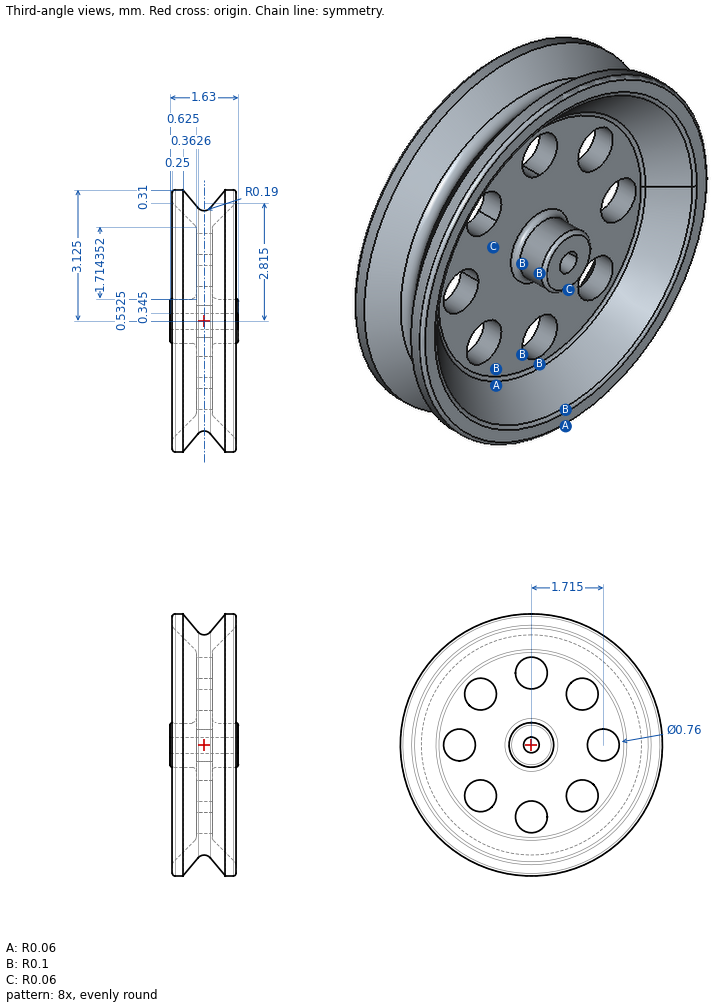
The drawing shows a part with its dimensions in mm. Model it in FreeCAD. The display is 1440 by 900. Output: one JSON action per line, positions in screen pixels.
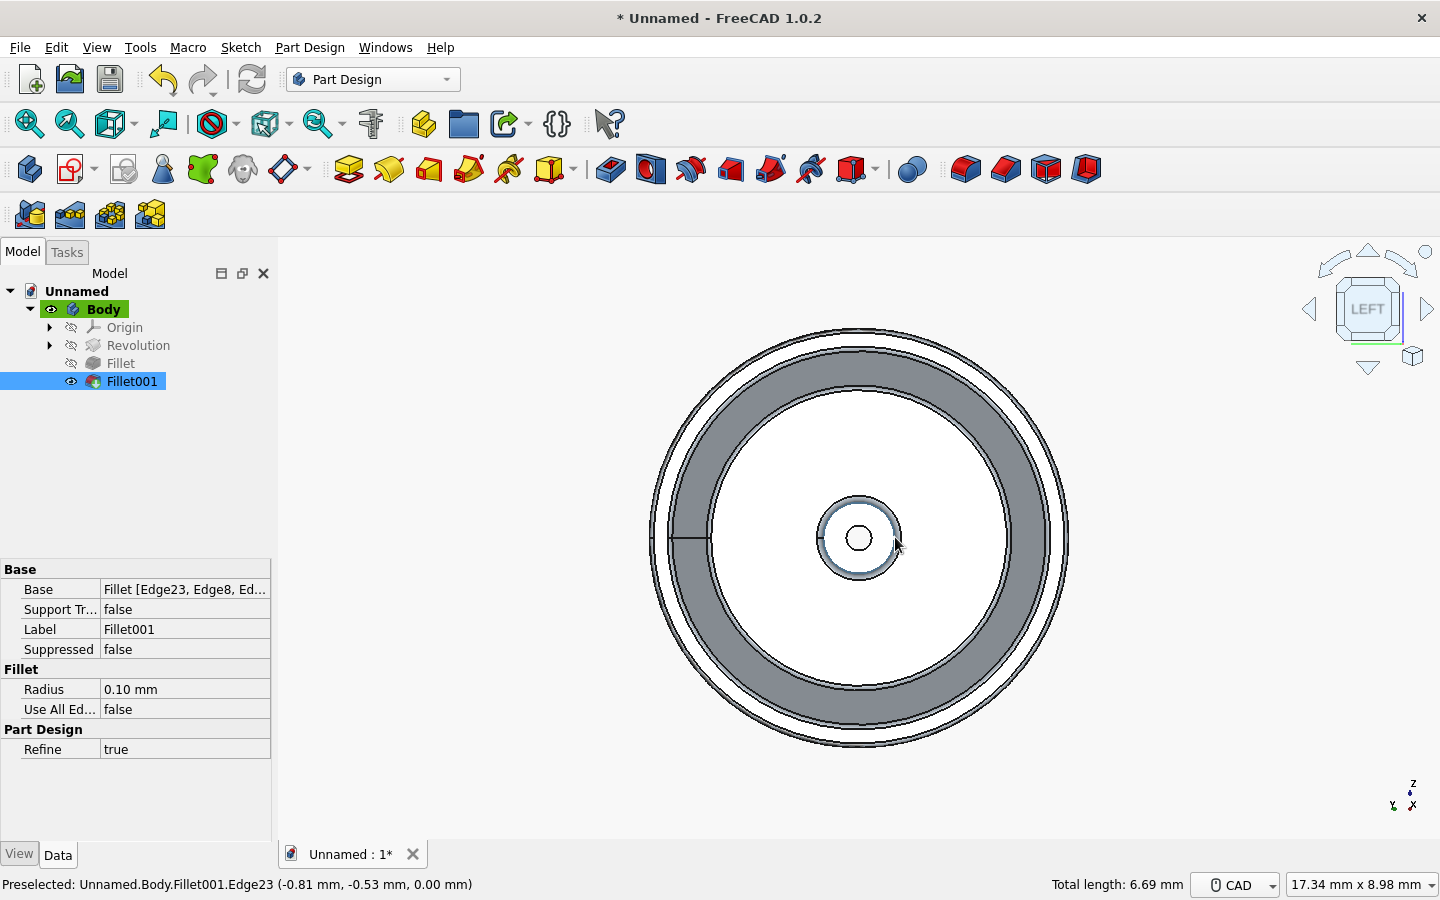
{"action": "left_click", "coordinate": [966, 170]}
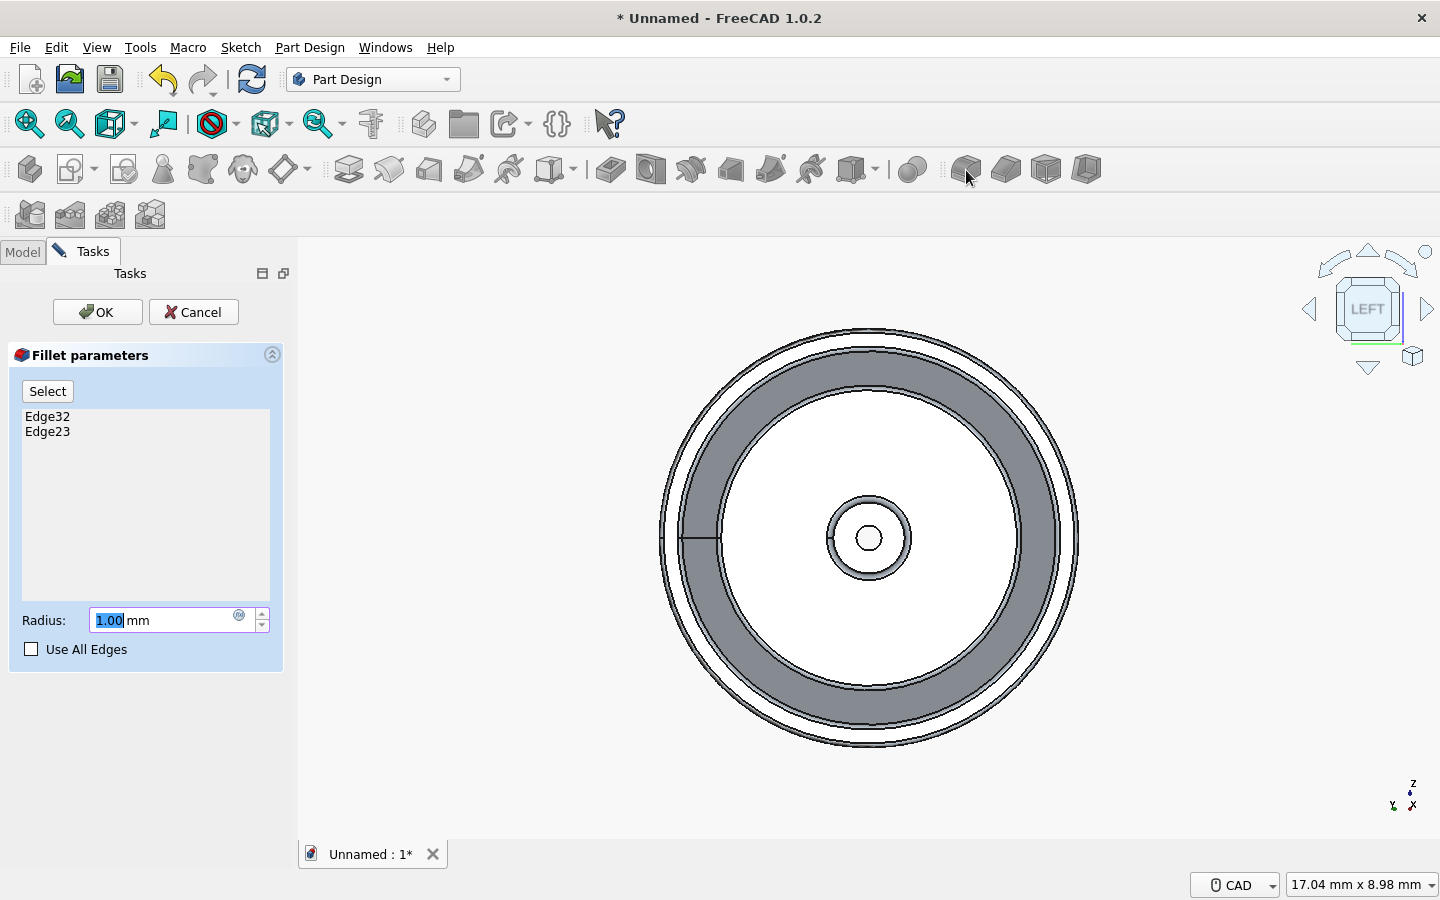
{"action": "type", "text": "0.06"}
{"action": "key", "text": "Tab"}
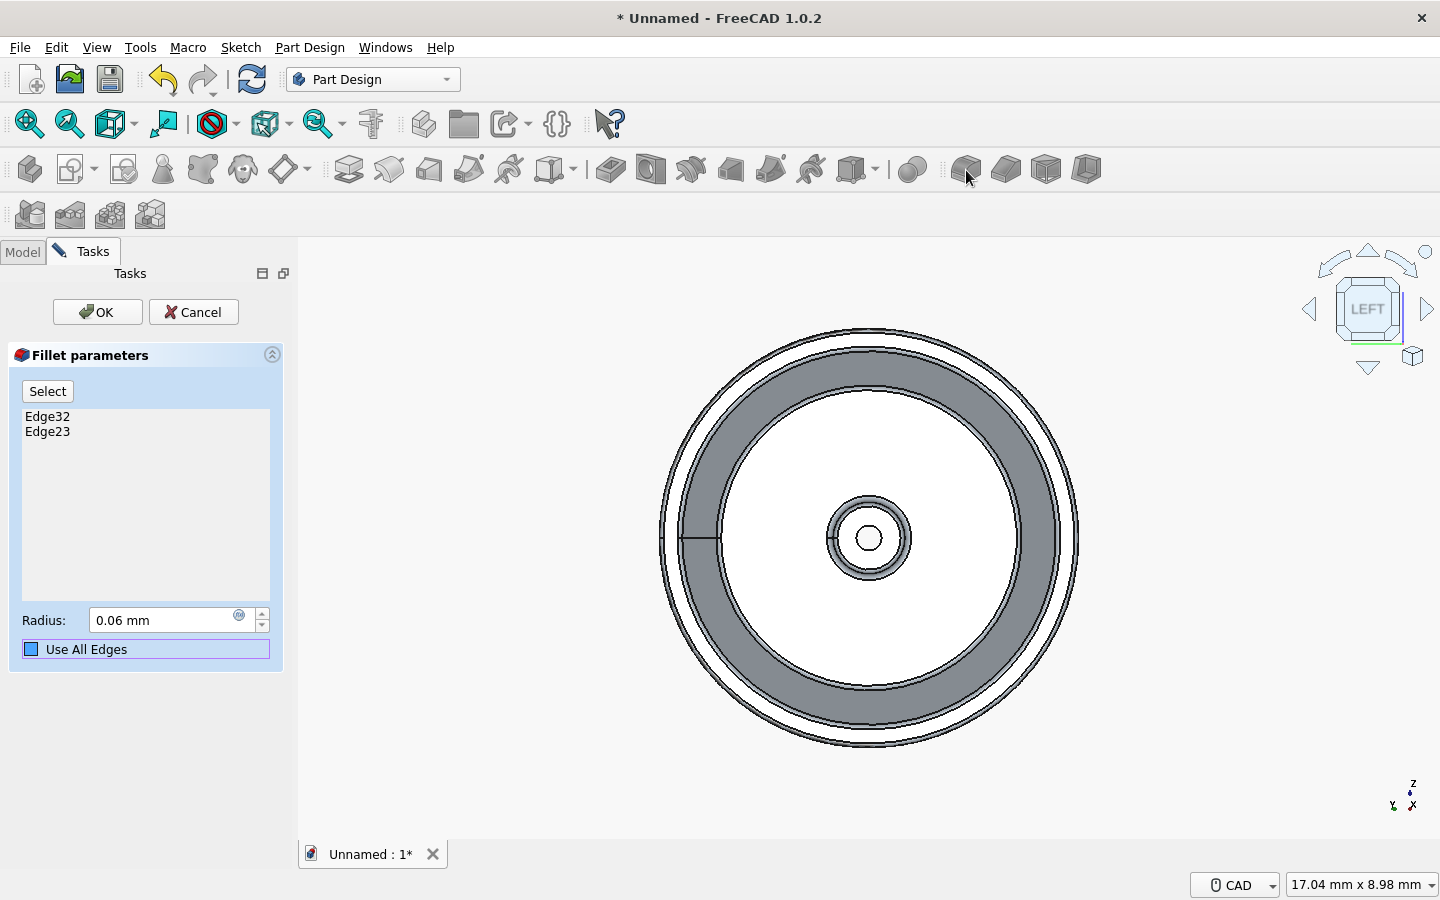
{"action": "left_click", "coordinate": [98, 312]}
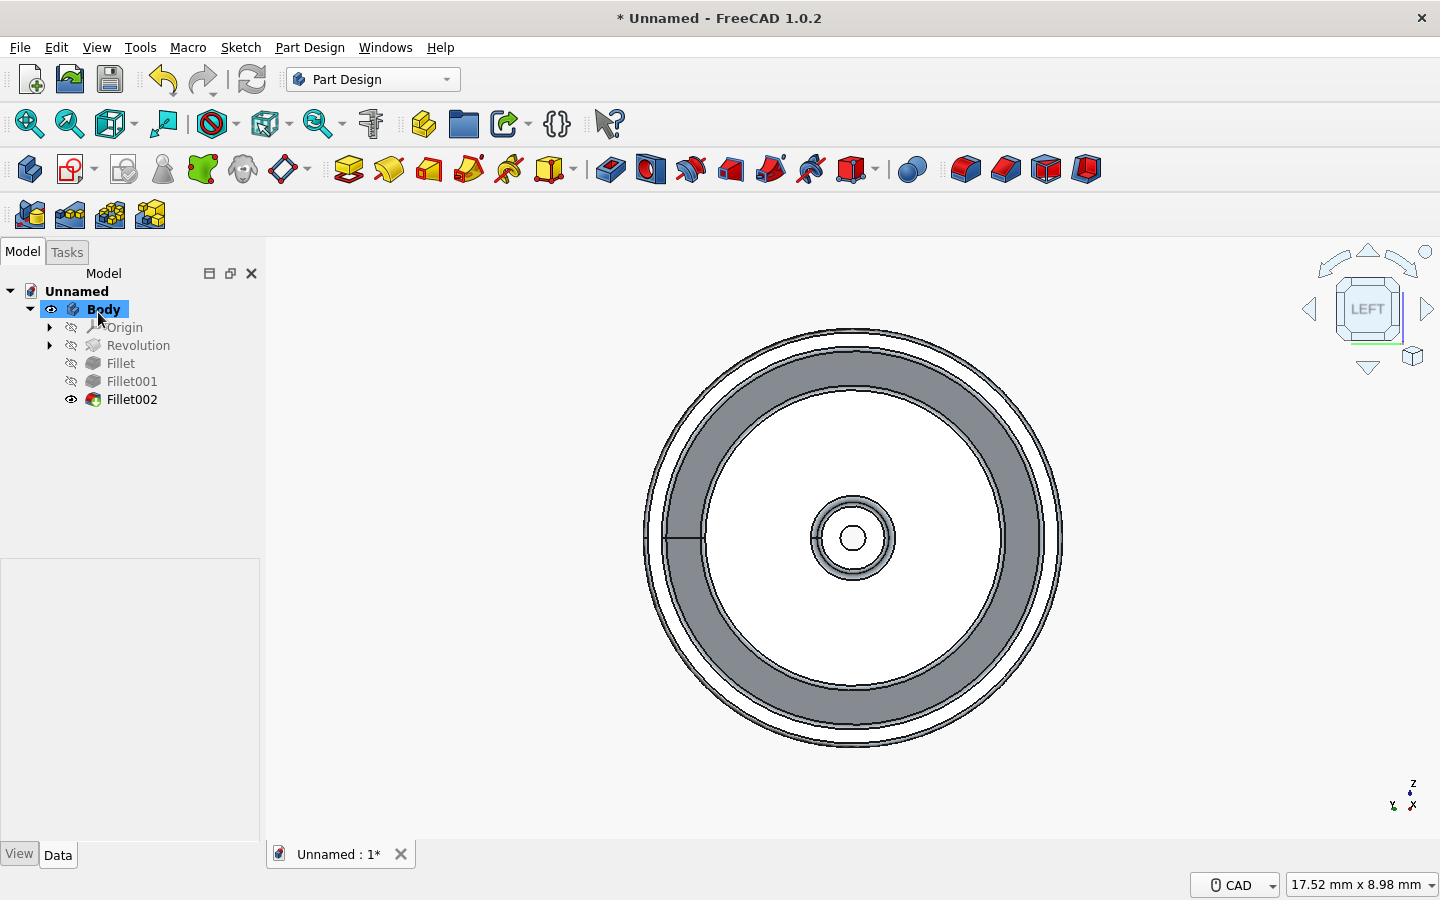
{"action": "left_click", "coordinate": [895, 453]}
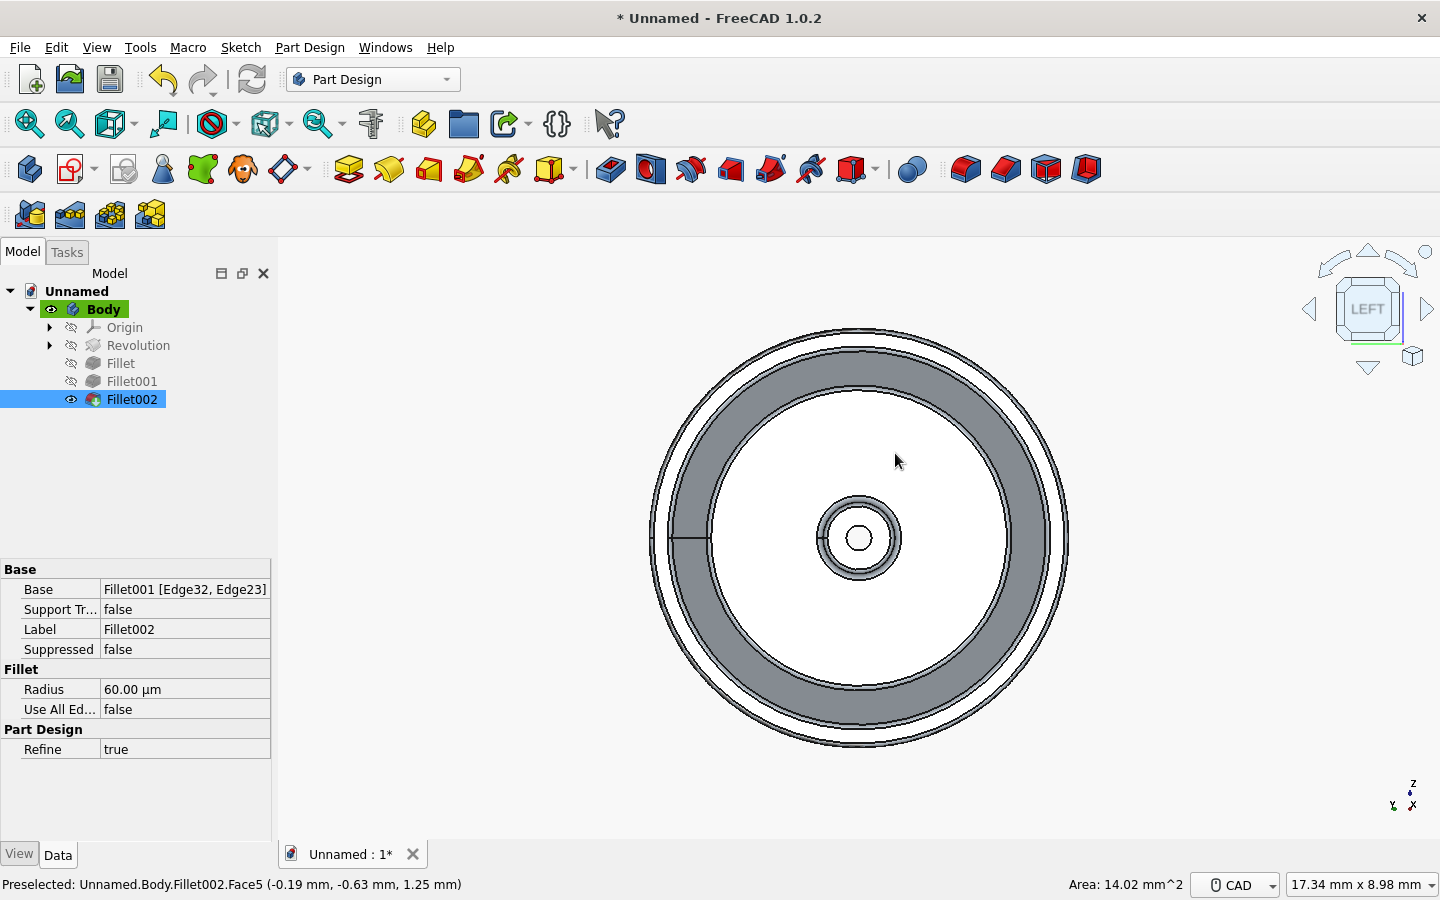
{"action": "left_click", "coordinate": [70, 170]}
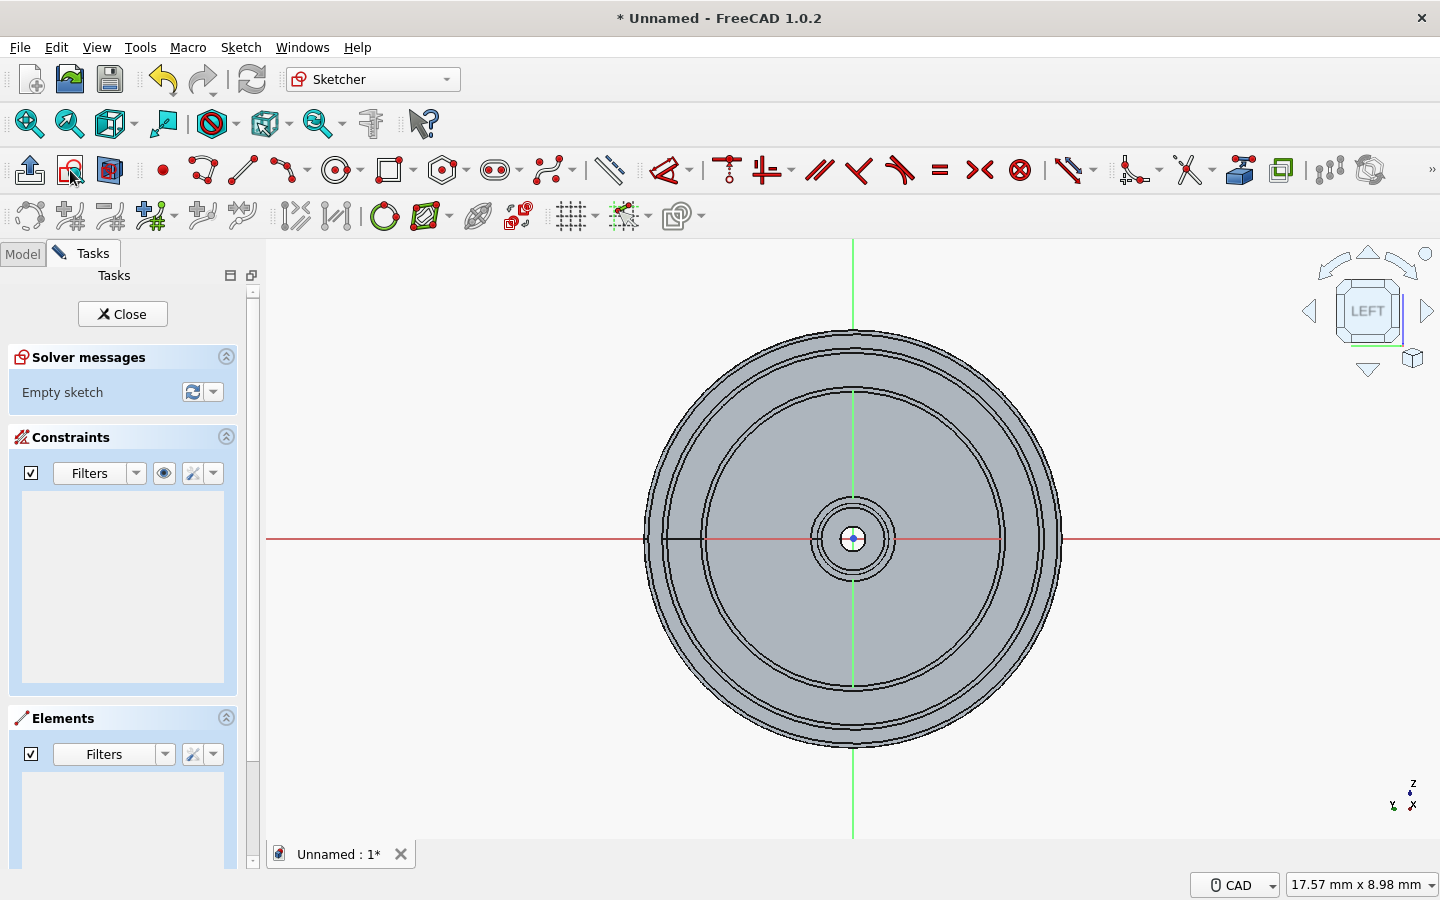
{"action": "left_click", "coordinate": [110, 170]}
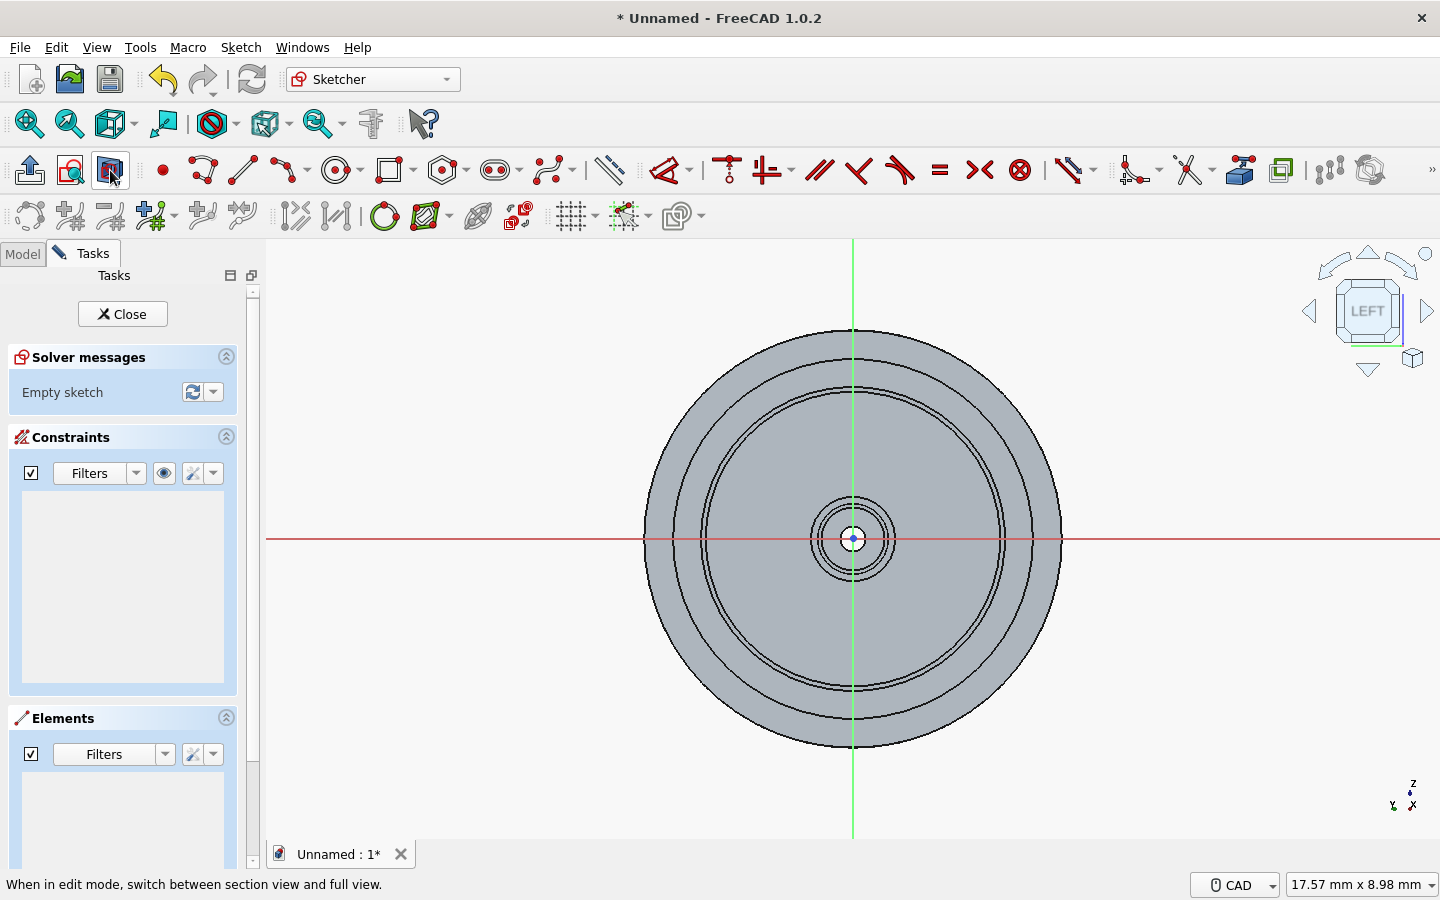
{"action": "scroll", "coordinate": [731, 539], "scroll_direction": "up", "scroll_amount": 10}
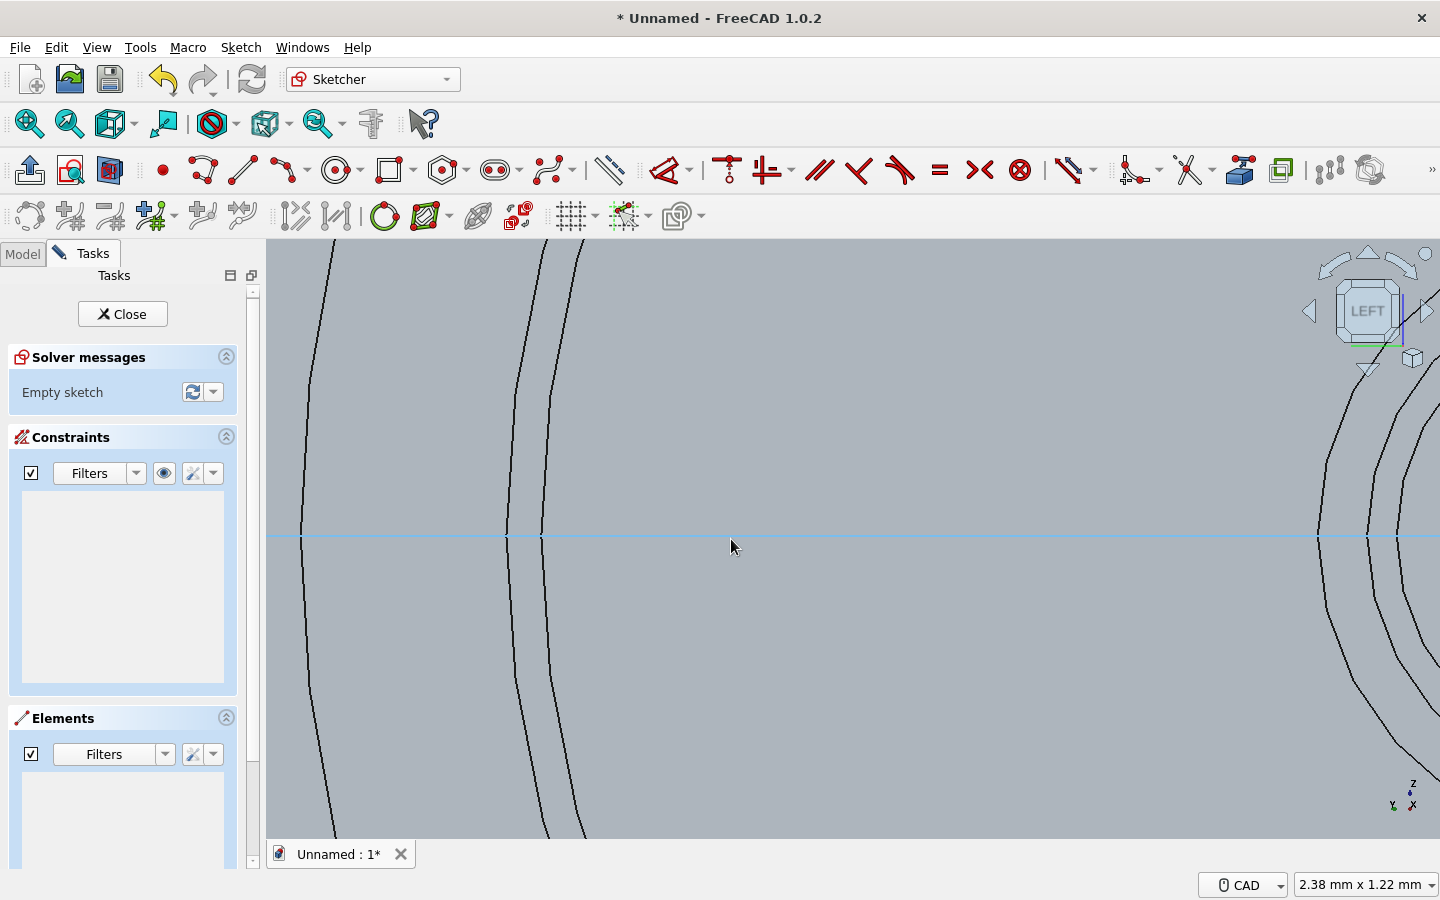
{"action": "left_click", "coordinate": [336, 170]}